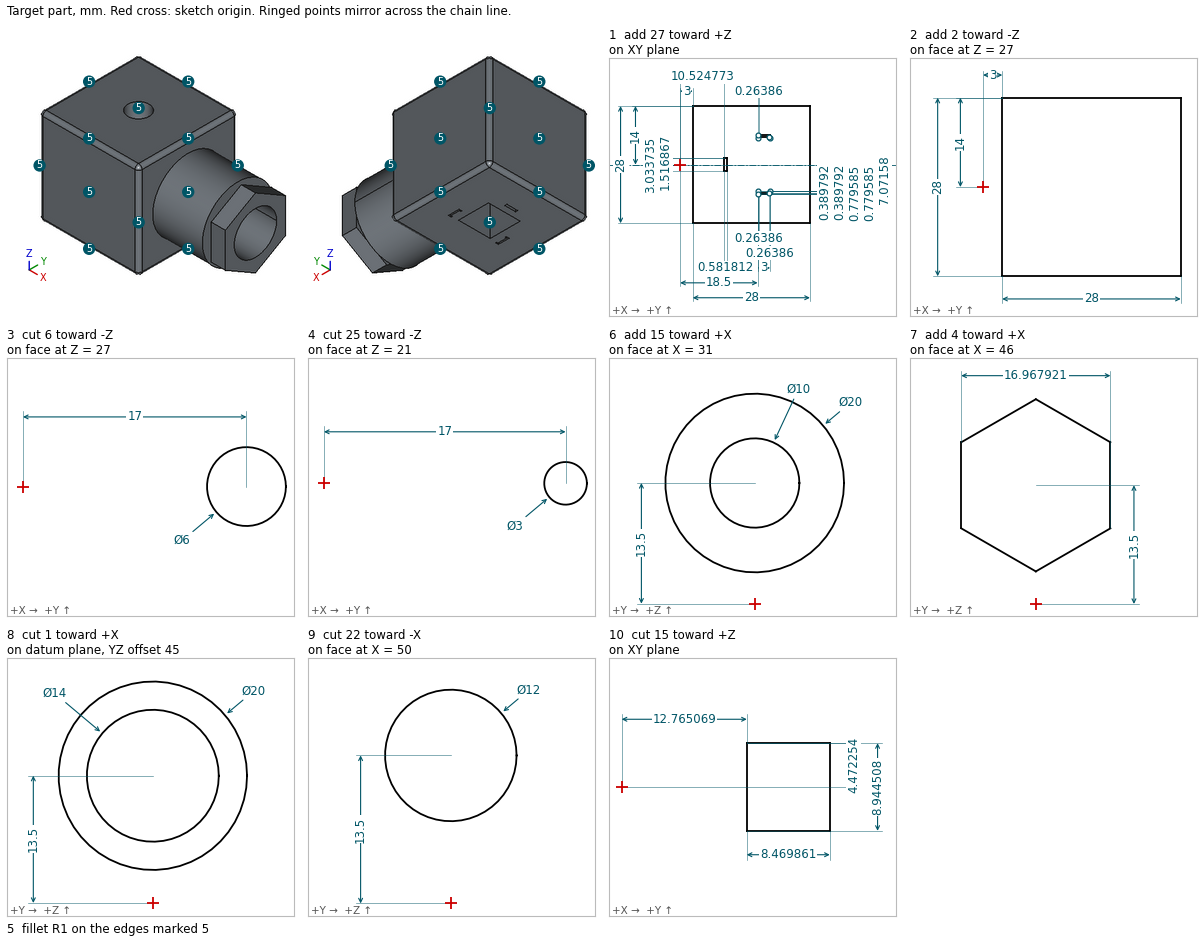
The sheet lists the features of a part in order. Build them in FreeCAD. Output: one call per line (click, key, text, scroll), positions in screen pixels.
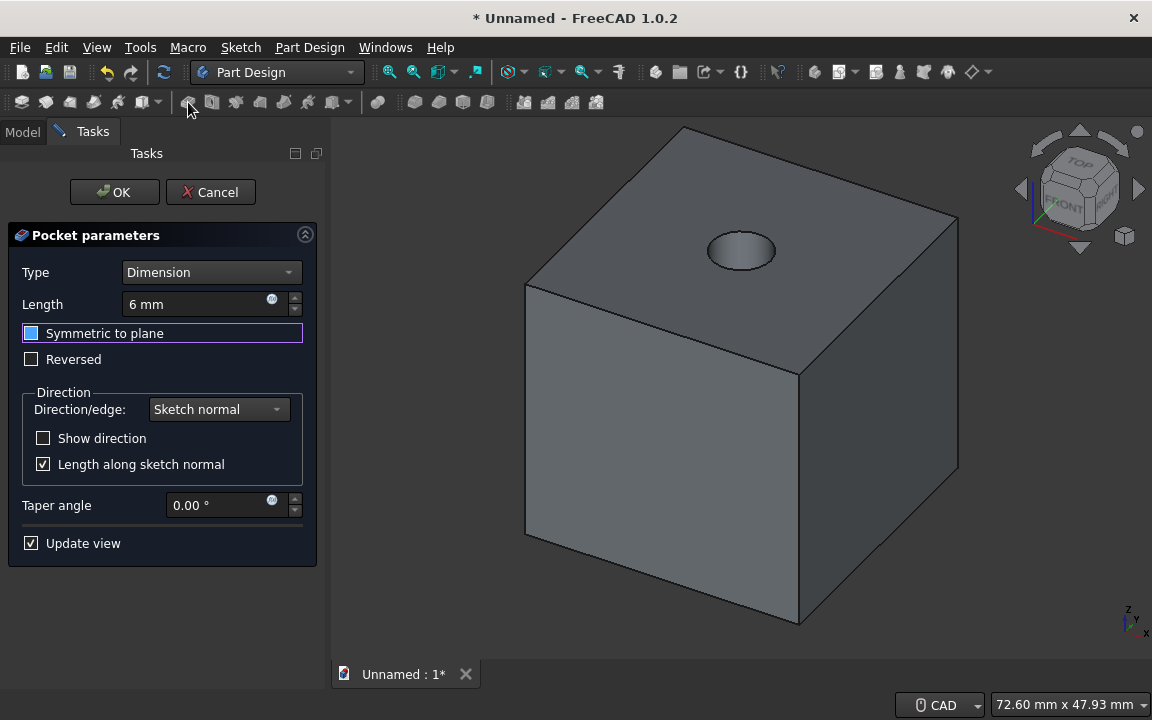
click(115, 192)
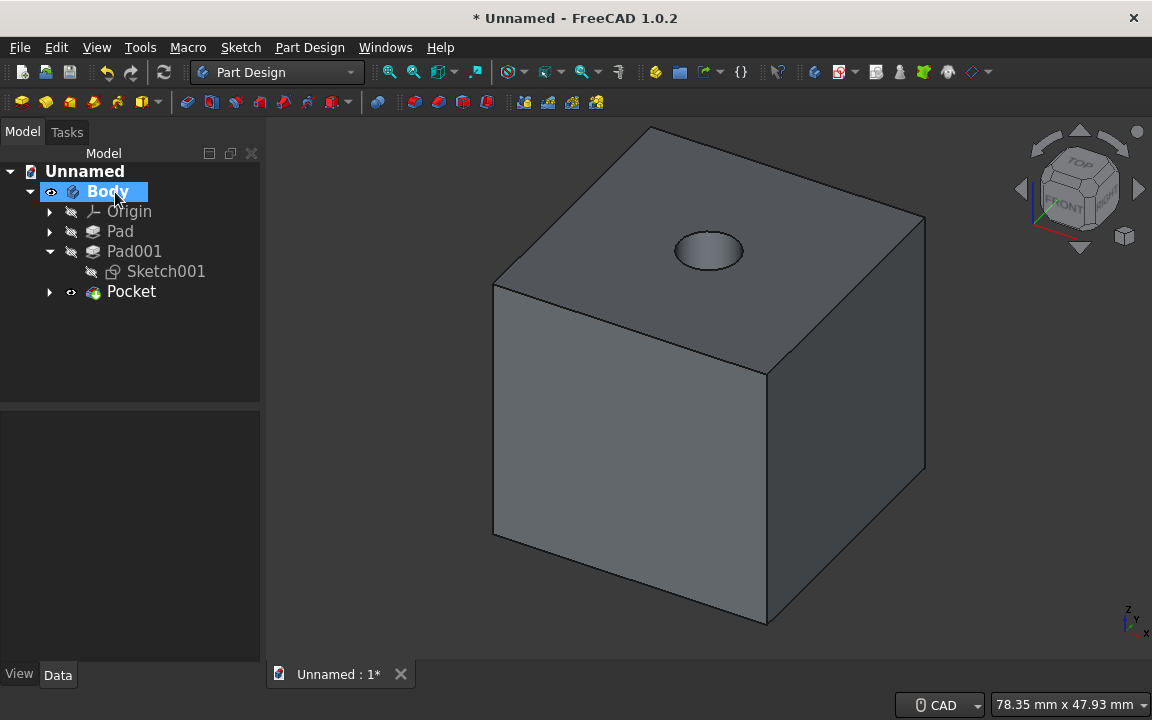
key(0)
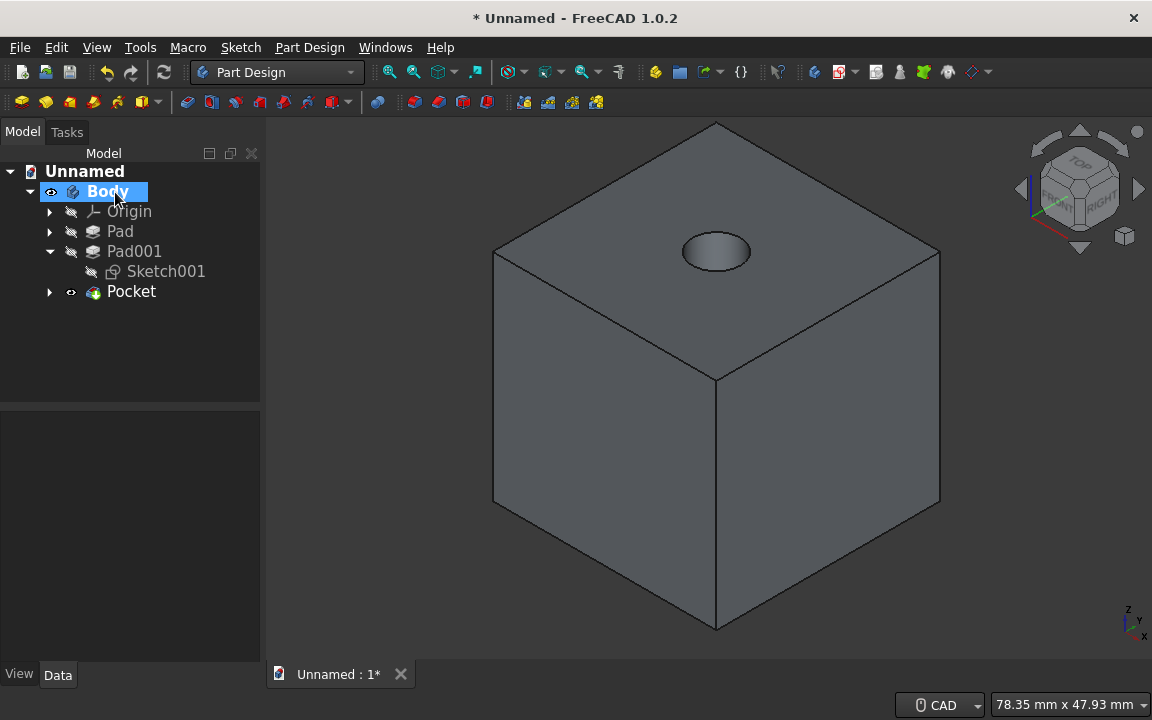
key(2)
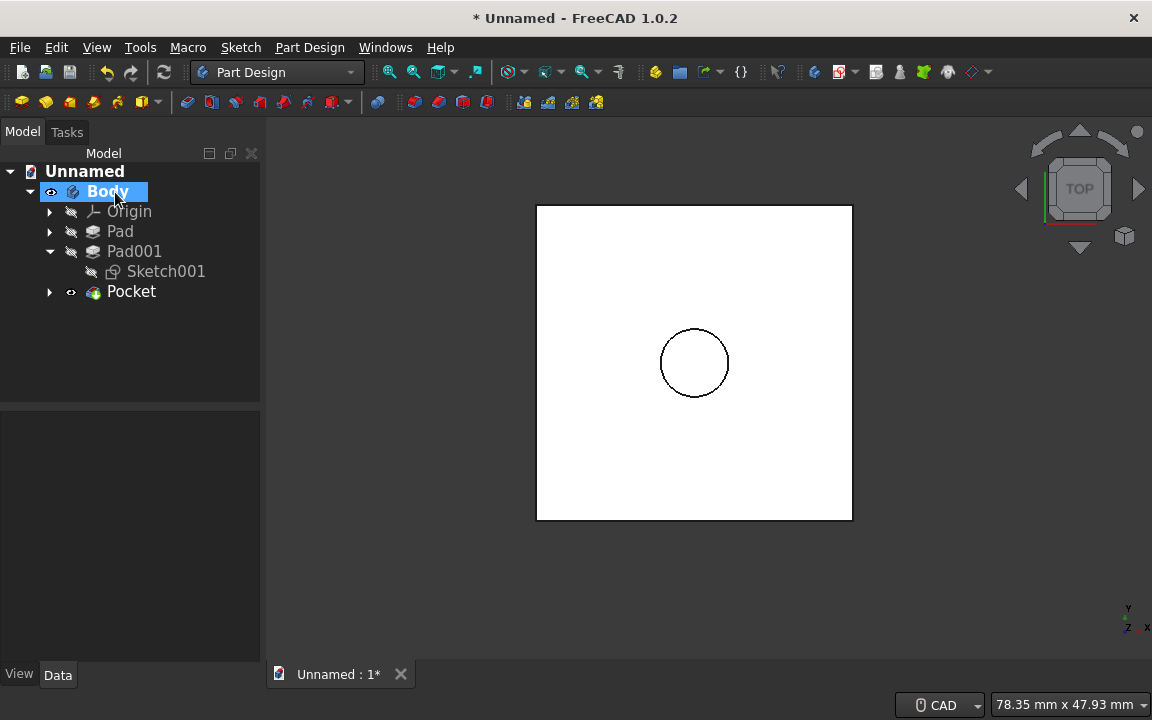
click(695, 362)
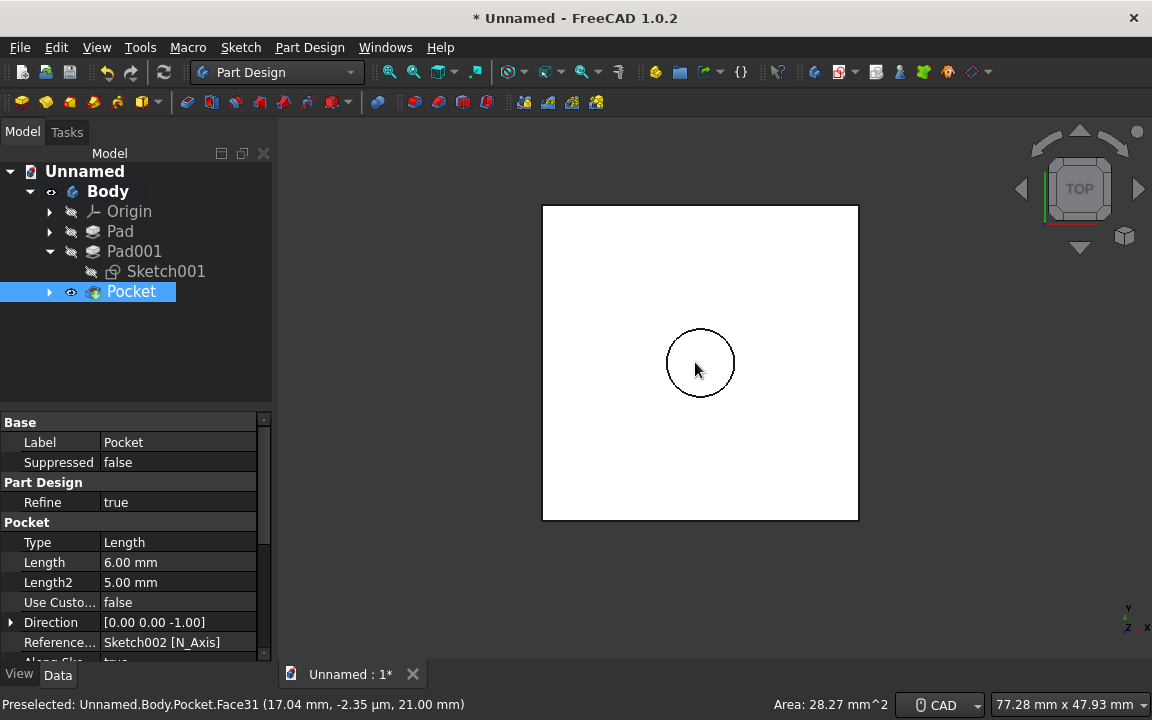
click(840, 72)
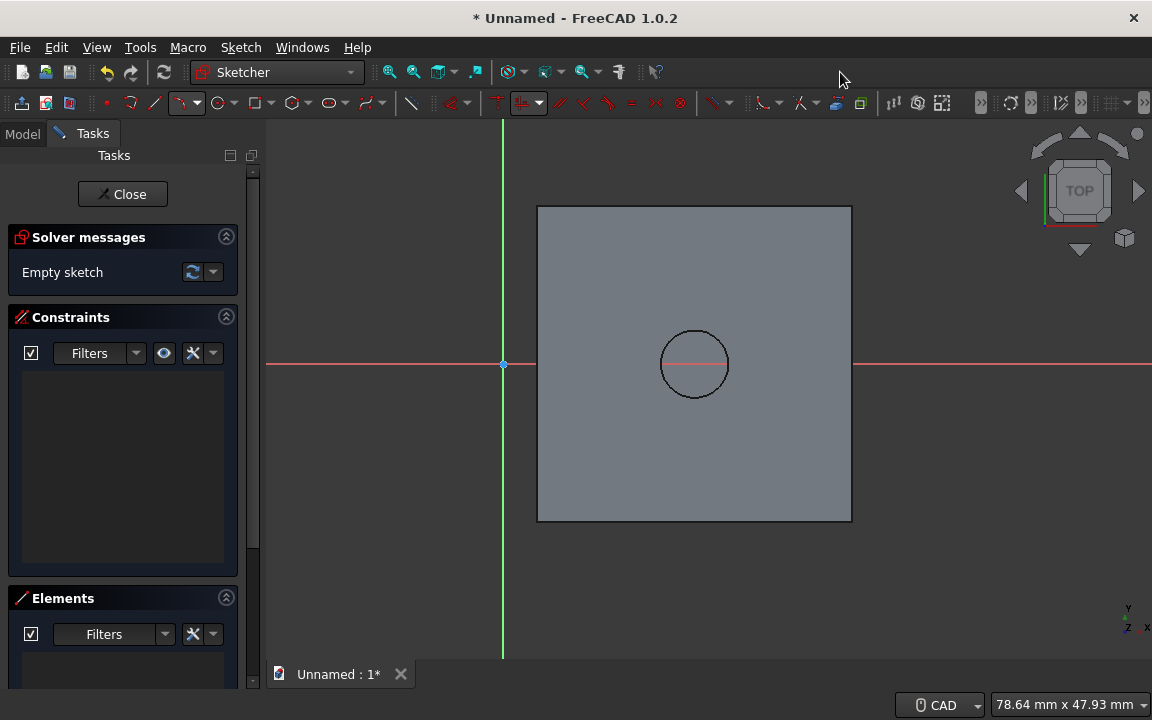
click(70, 104)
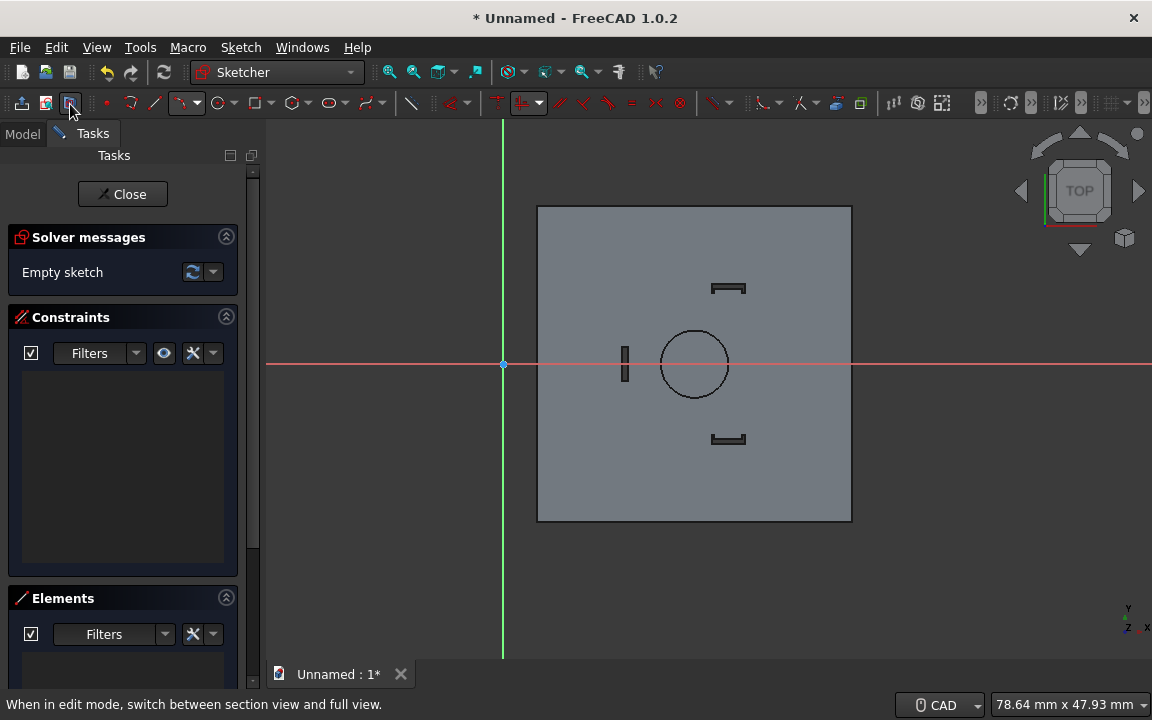
scroll(700, 362, up, 12)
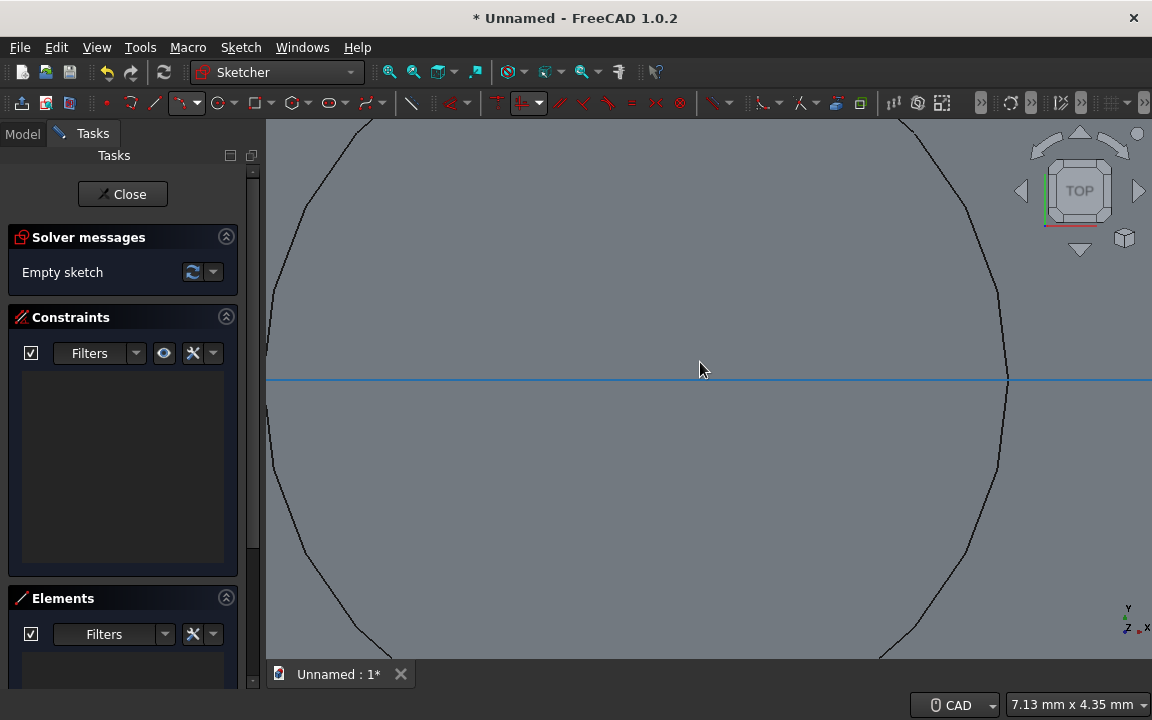
click(218, 104)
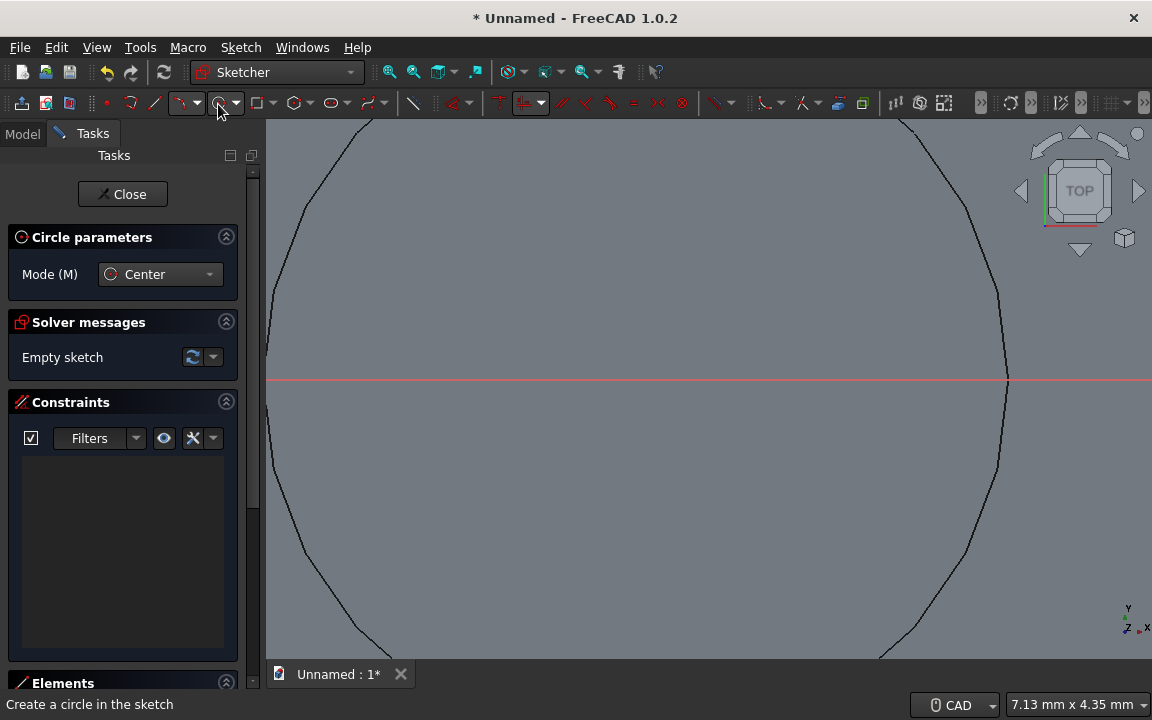
click(636, 380)
click(767, 249)
key(Escape)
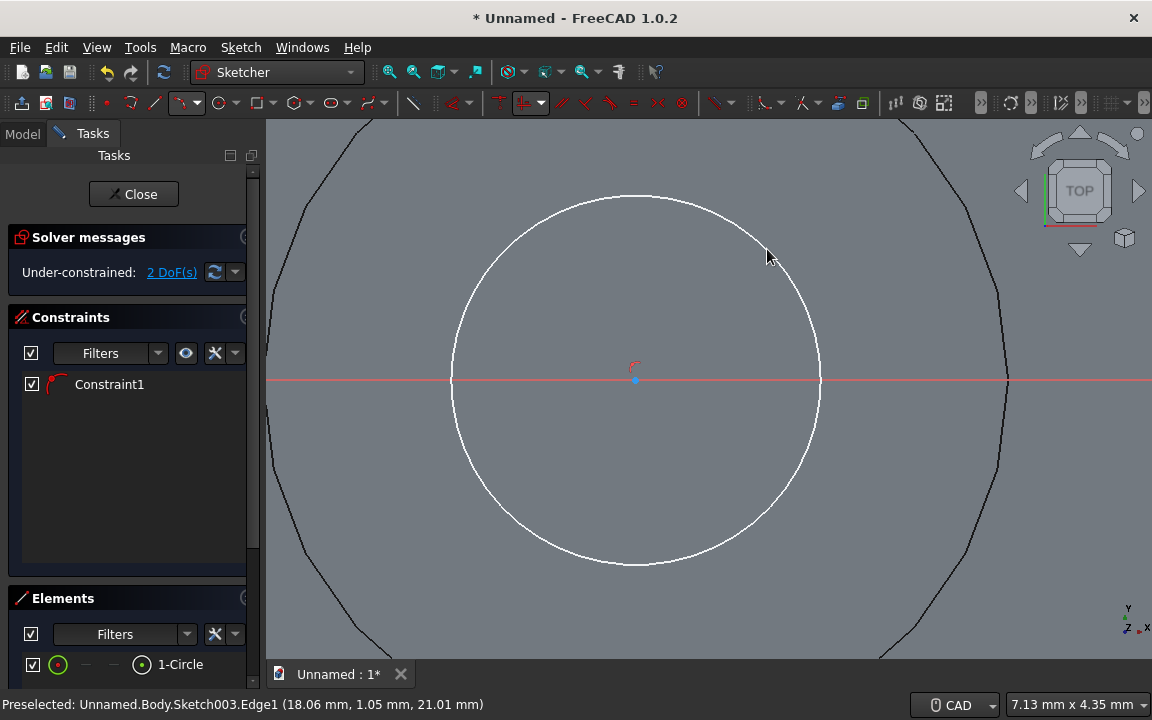
click(452, 104)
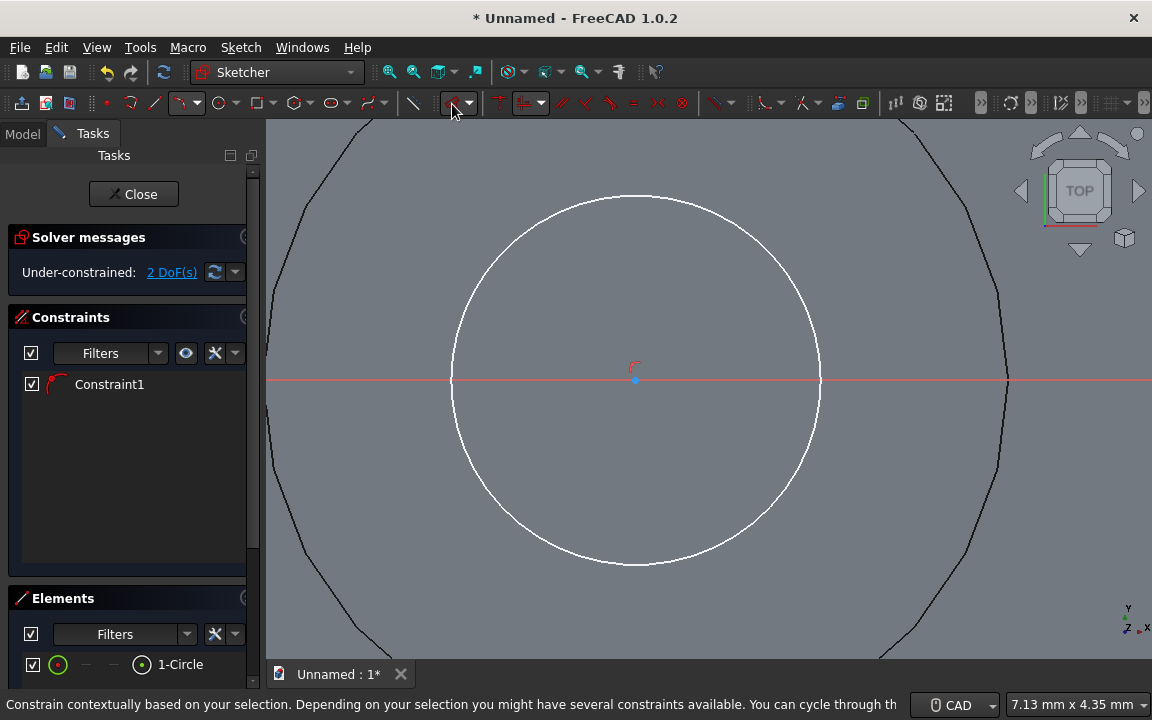
click(766, 249)
click(789, 226)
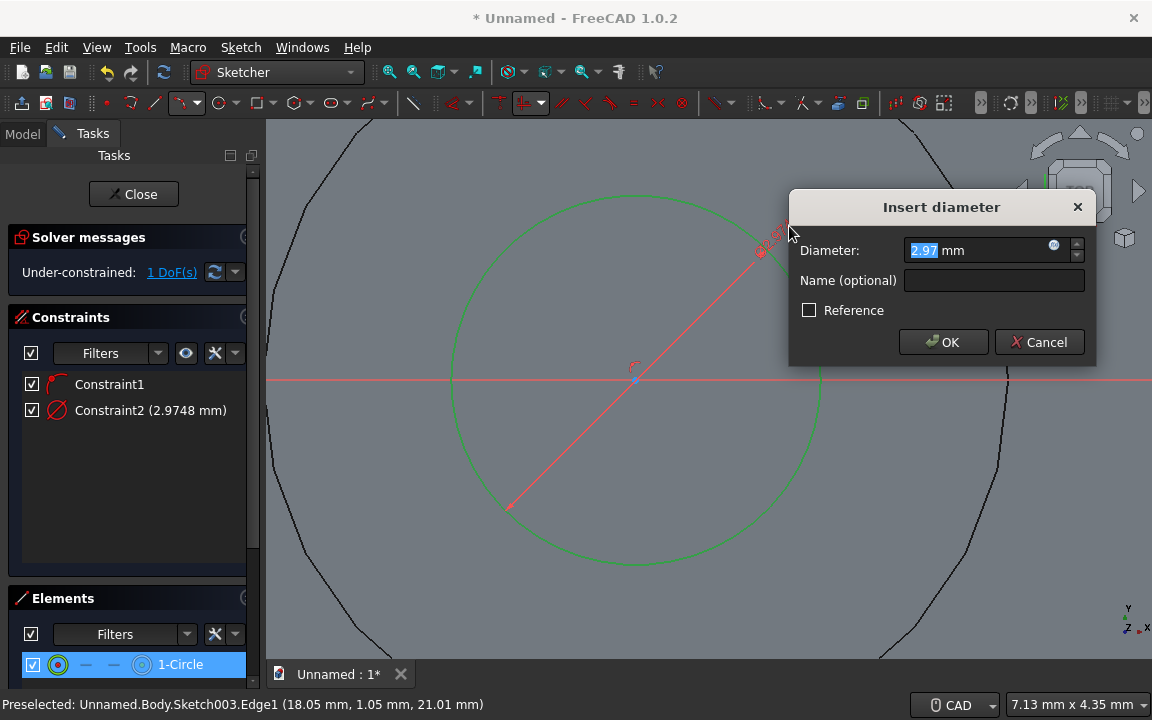
text(3)
key(Return)